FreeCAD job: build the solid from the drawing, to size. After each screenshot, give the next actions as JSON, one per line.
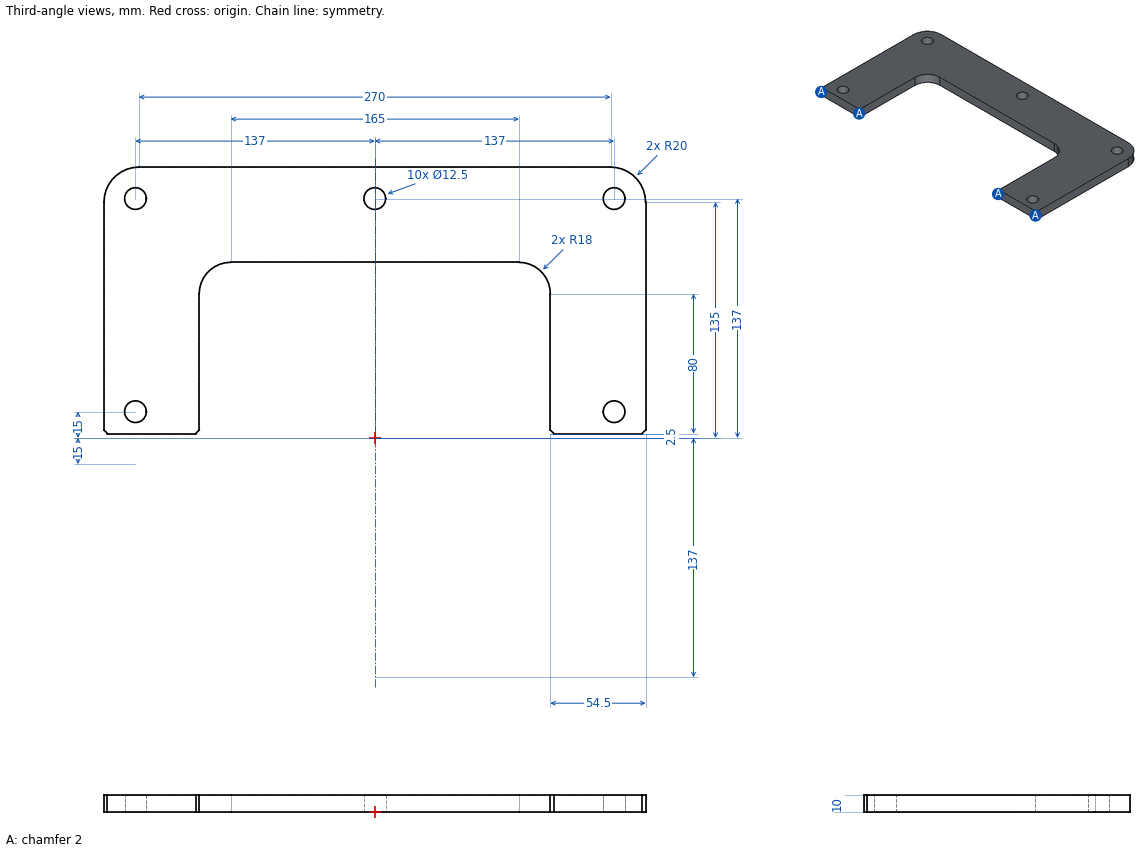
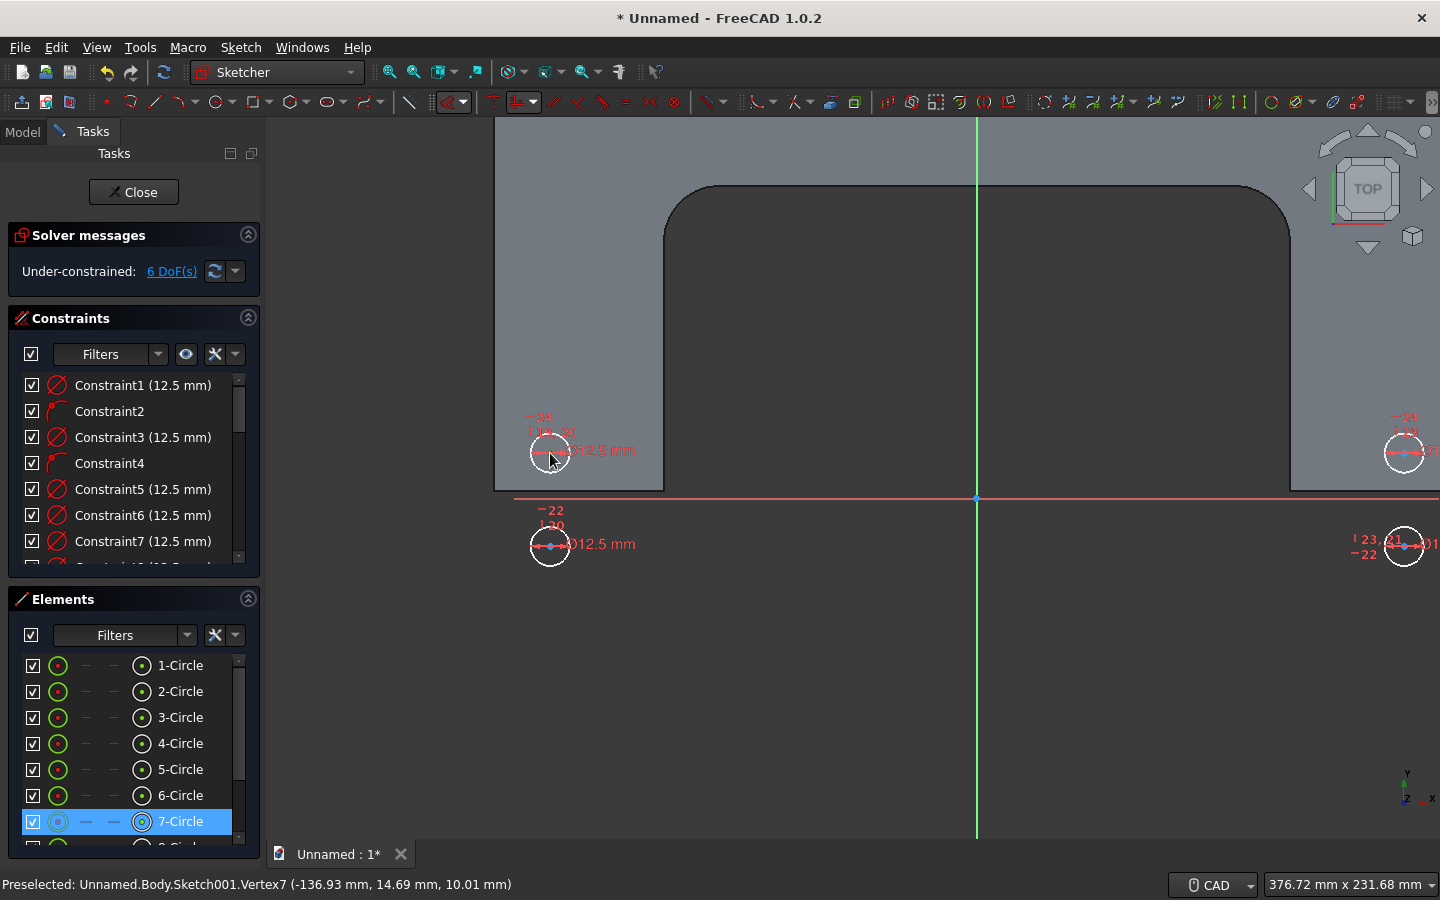
{"action": "key", "text": "i"}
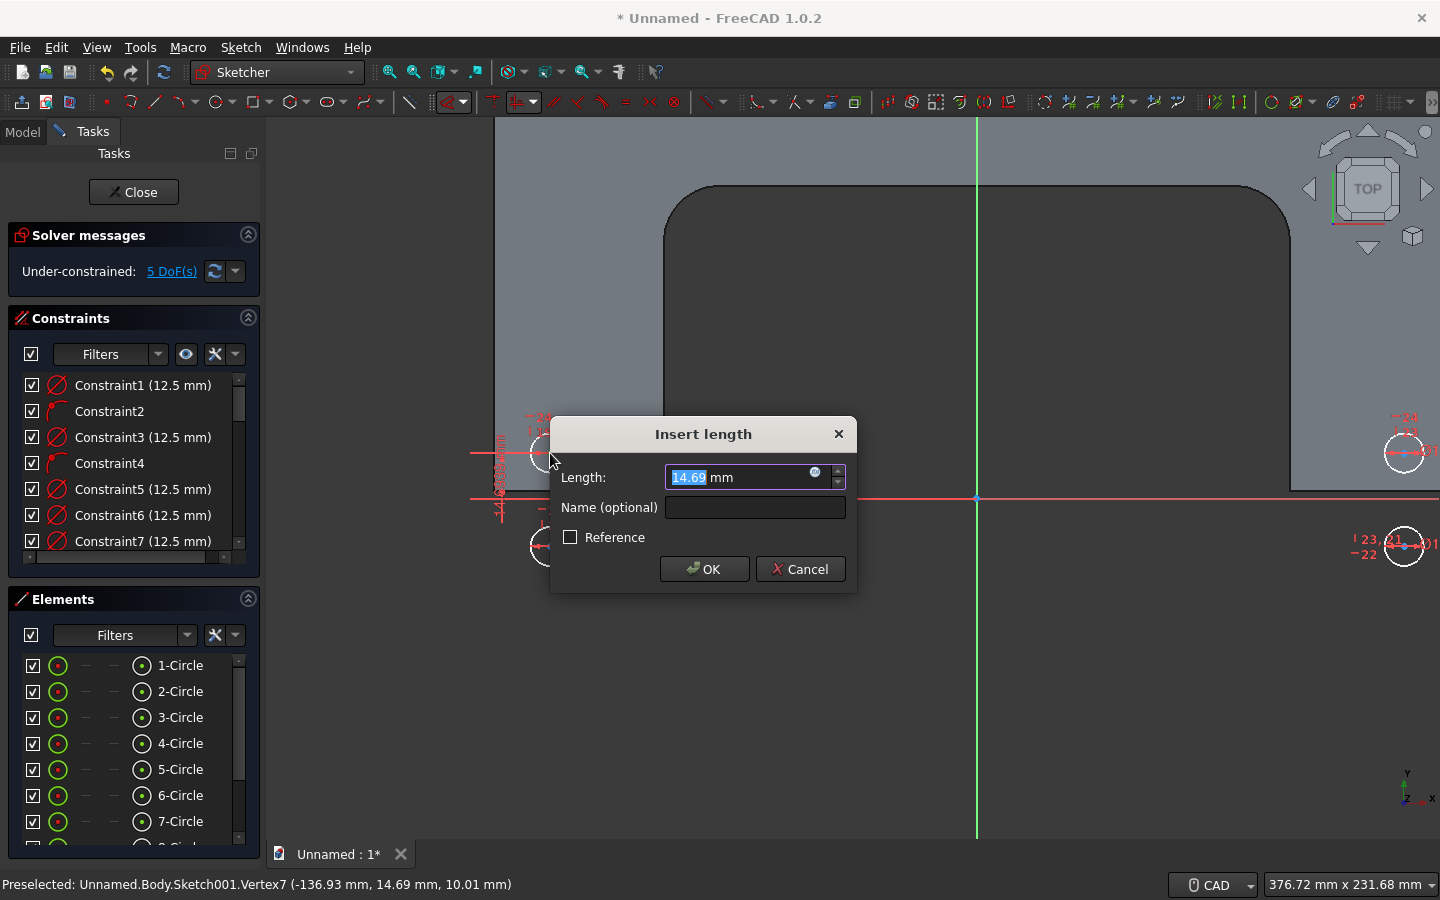
{"action": "type", "text": "15"}
{"action": "key", "text": "Return"}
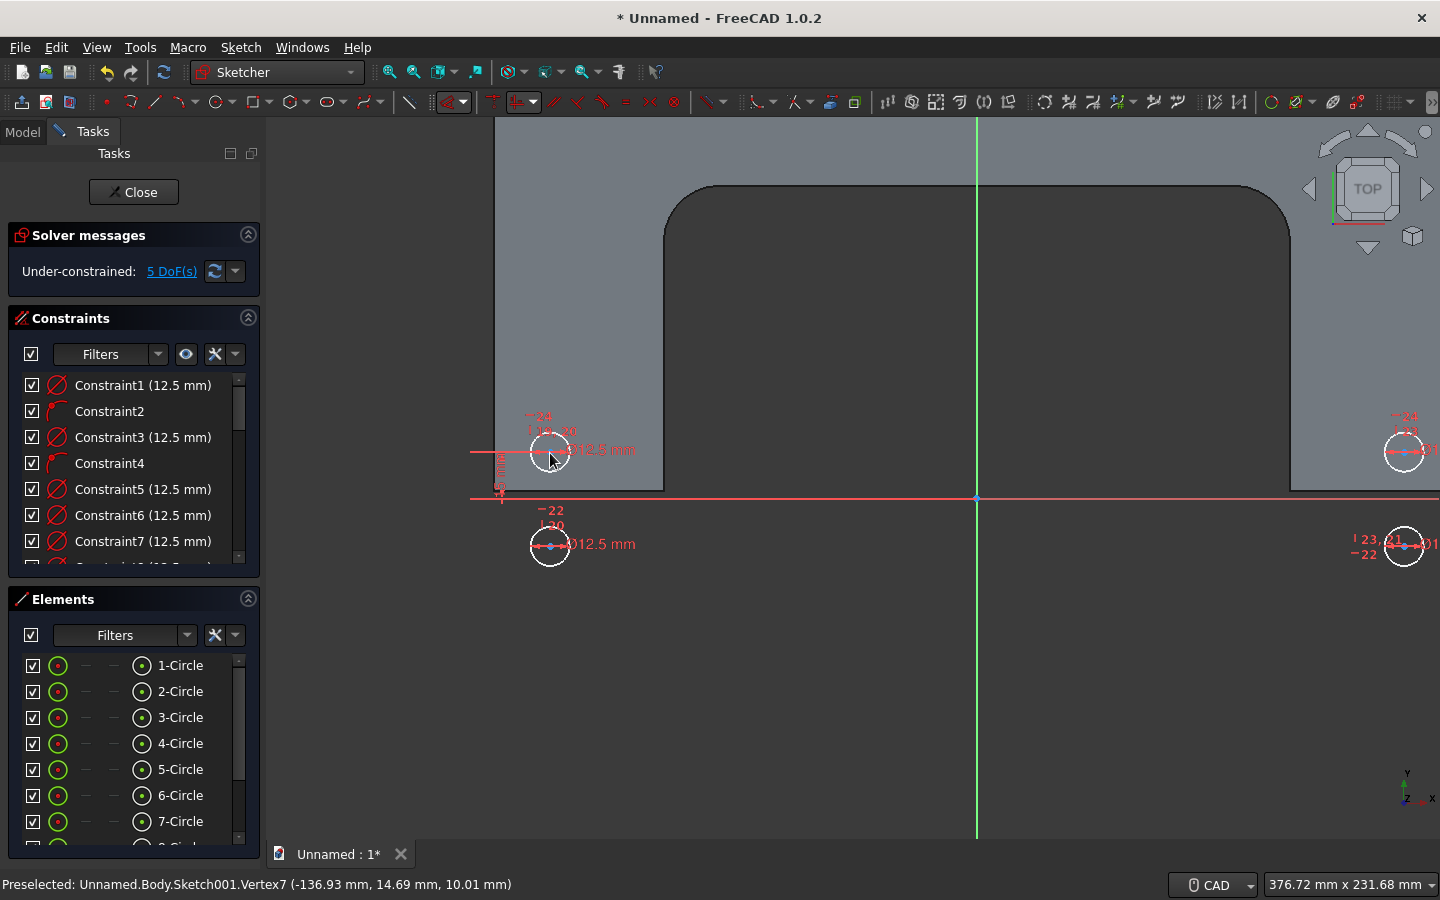
{"action": "left_click", "coordinate": [550, 546]}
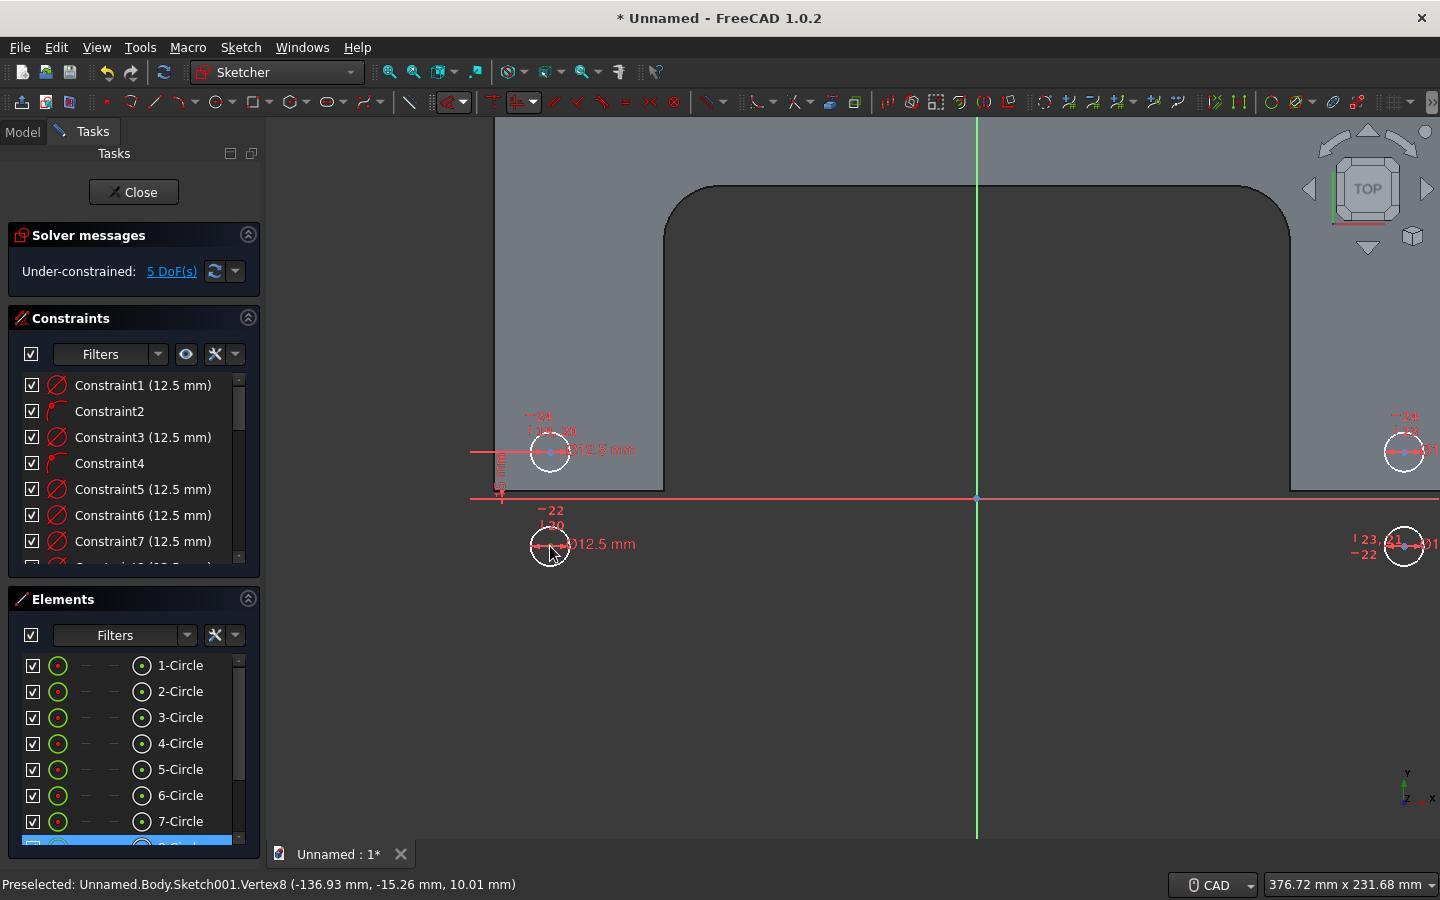
{"action": "key", "text": "i"}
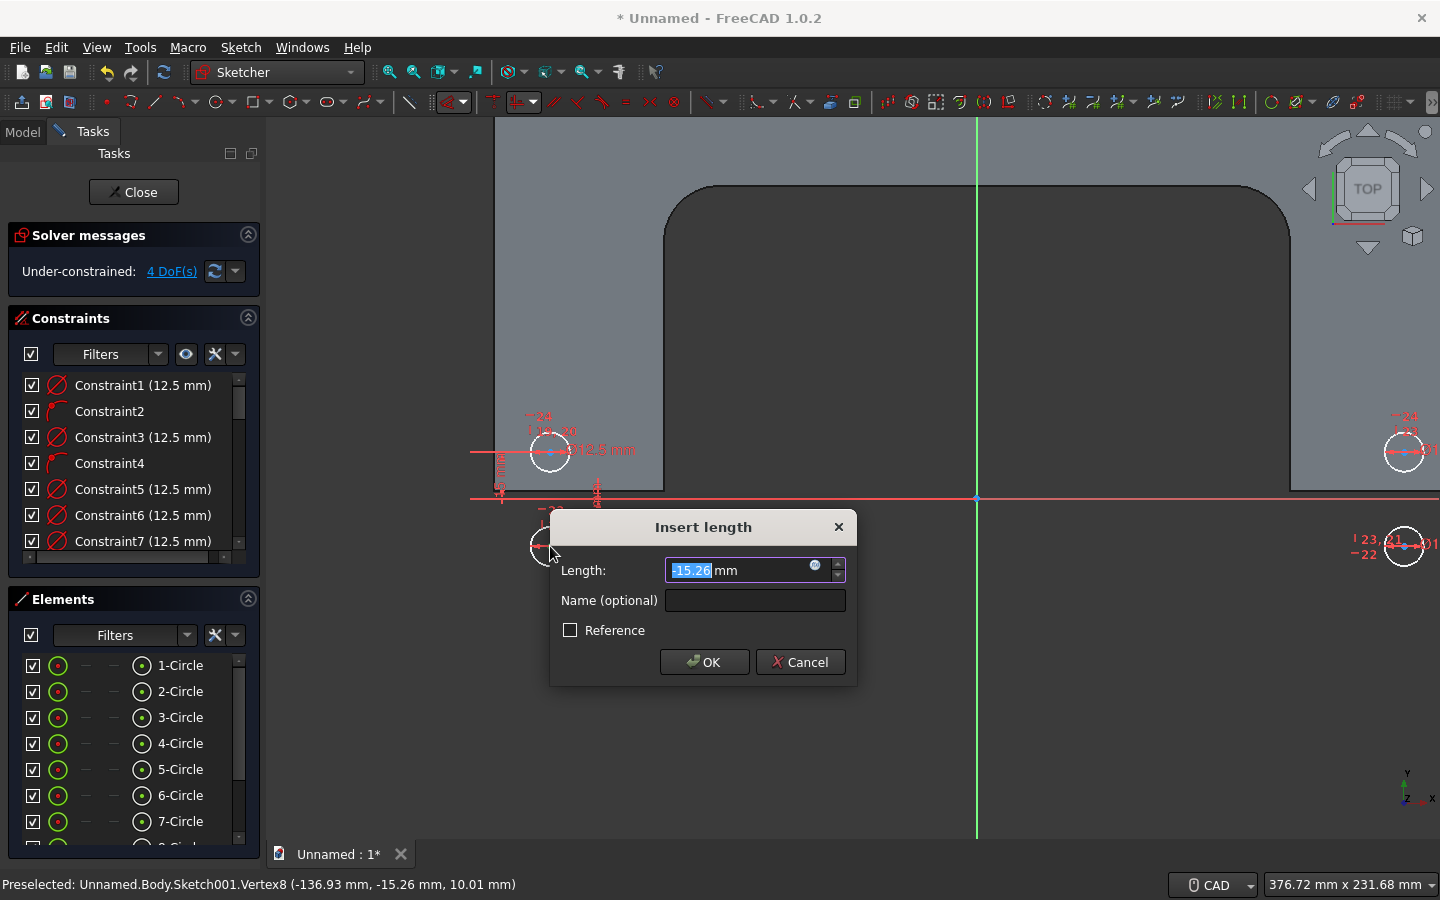
{"action": "type", "text": "-15"}
{"action": "key", "text": "Return"}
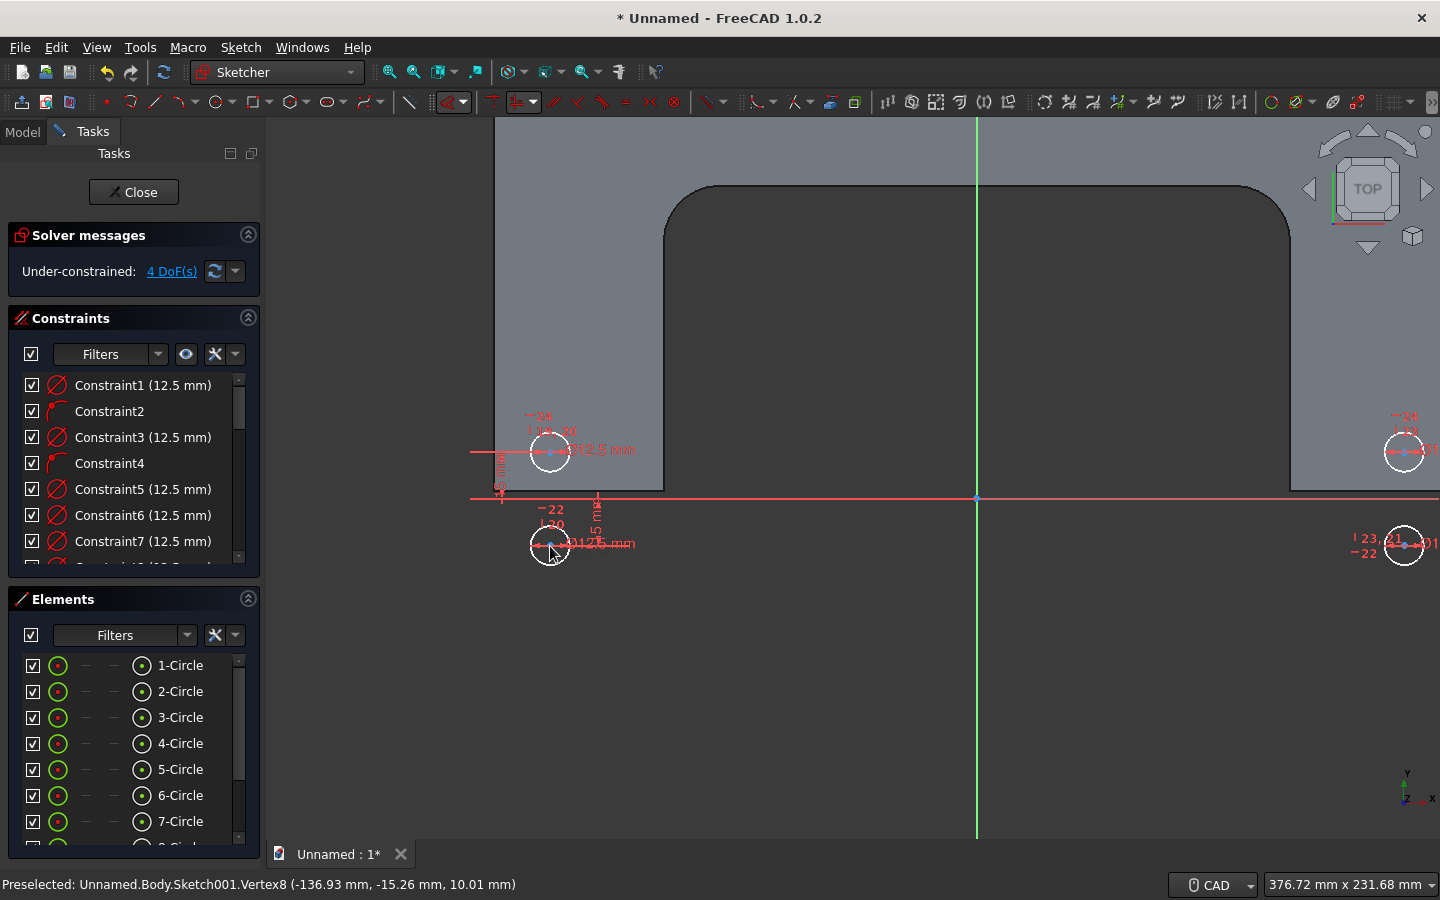
{"action": "scroll", "coordinate": [550, 453], "scroll_direction": "down", "scroll_amount": 3}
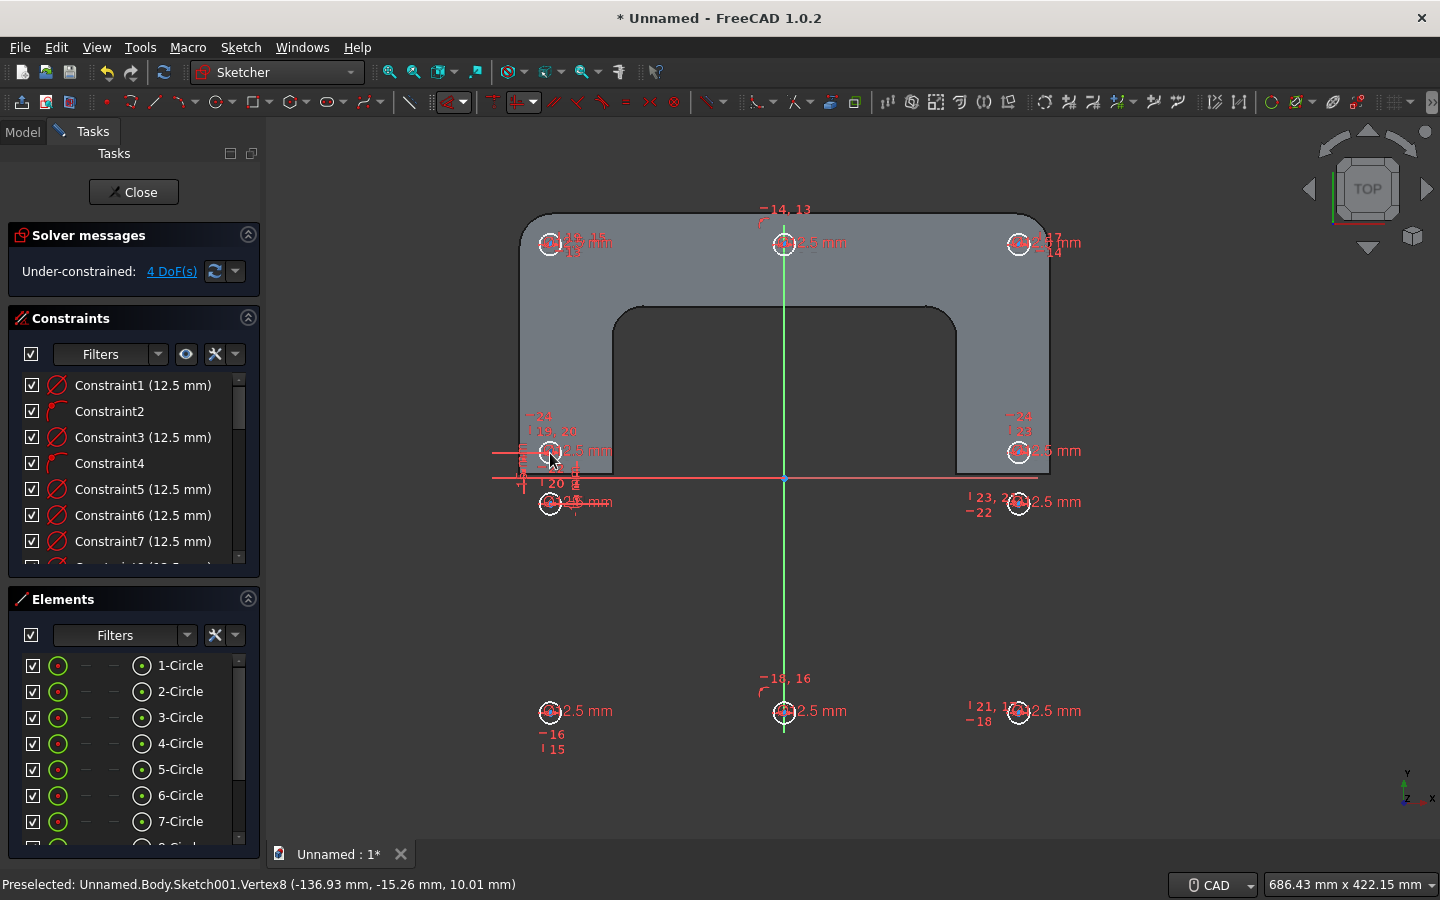
{"action": "left_click", "coordinate": [784, 245]}